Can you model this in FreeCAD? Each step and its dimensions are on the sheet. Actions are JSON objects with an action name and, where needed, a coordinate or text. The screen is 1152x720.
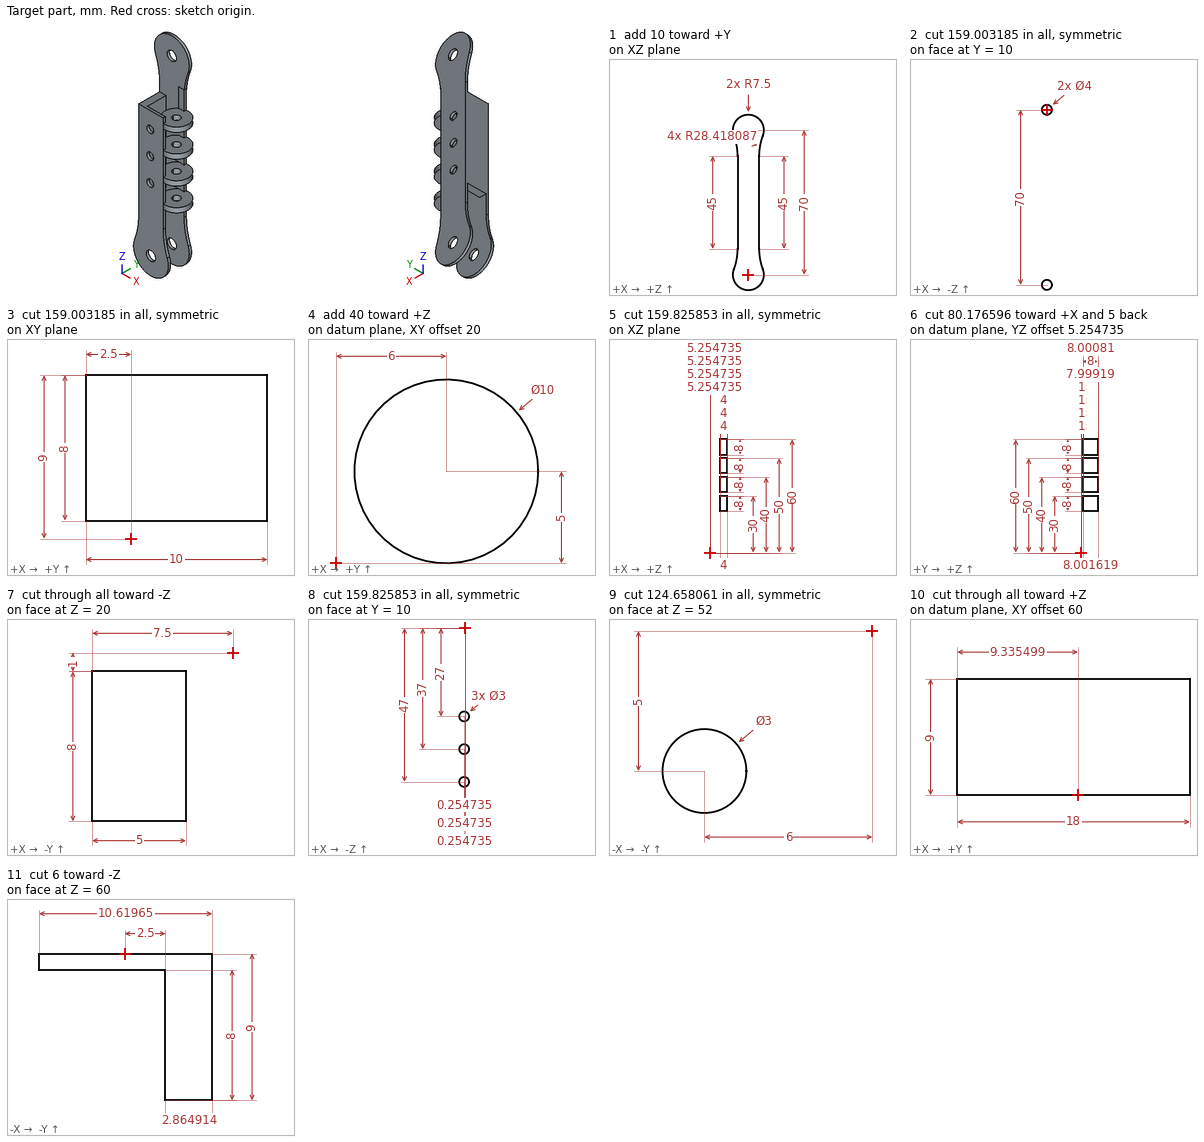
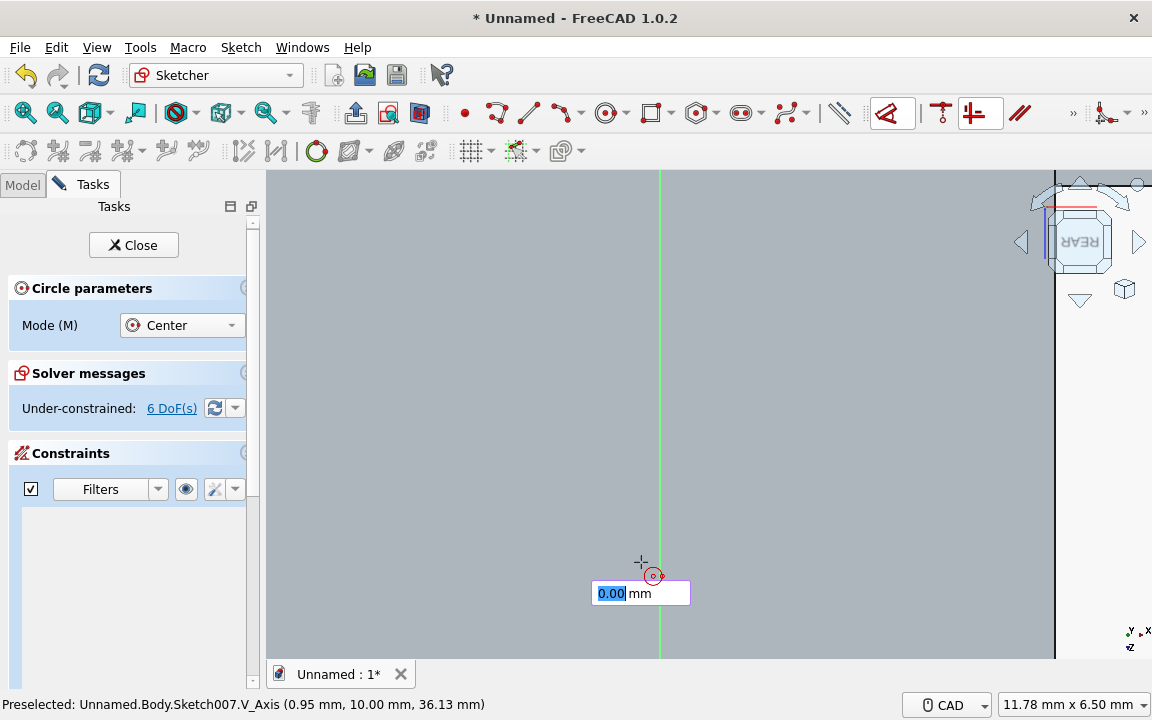
{"action": "scroll", "coordinate": [640, 570], "scroll_direction": "down", "scroll_amount": 12}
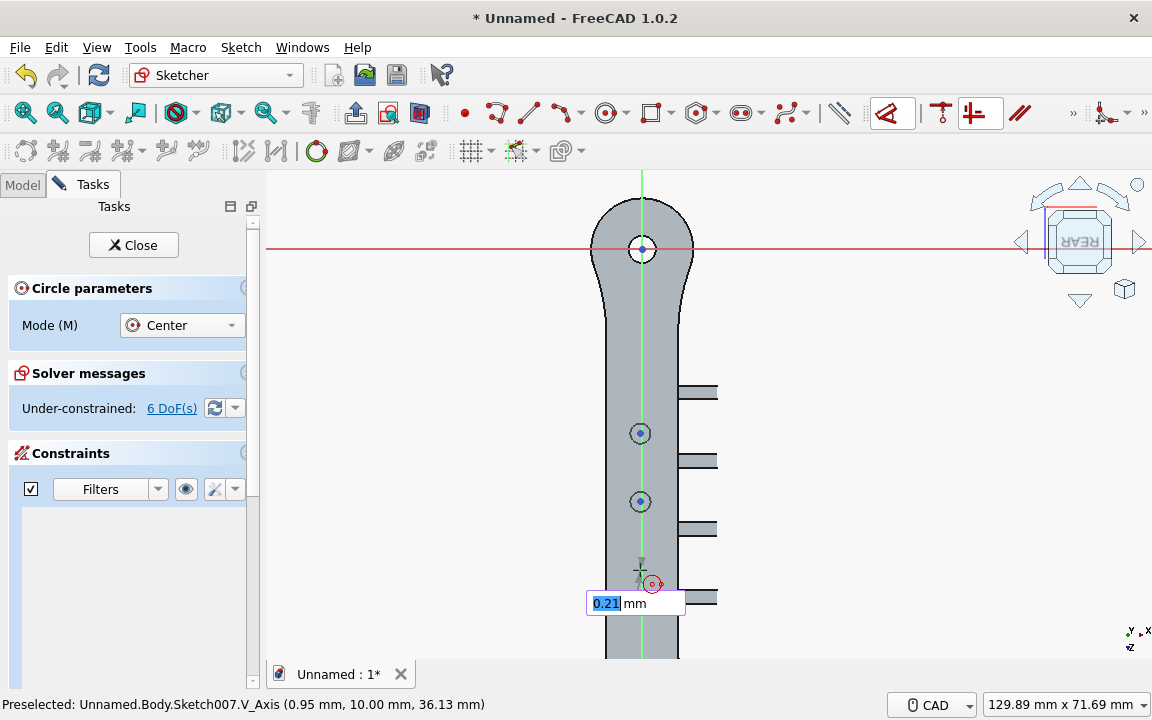
{"action": "scroll", "coordinate": [648, 563], "scroll_direction": "up", "scroll_amount": 6}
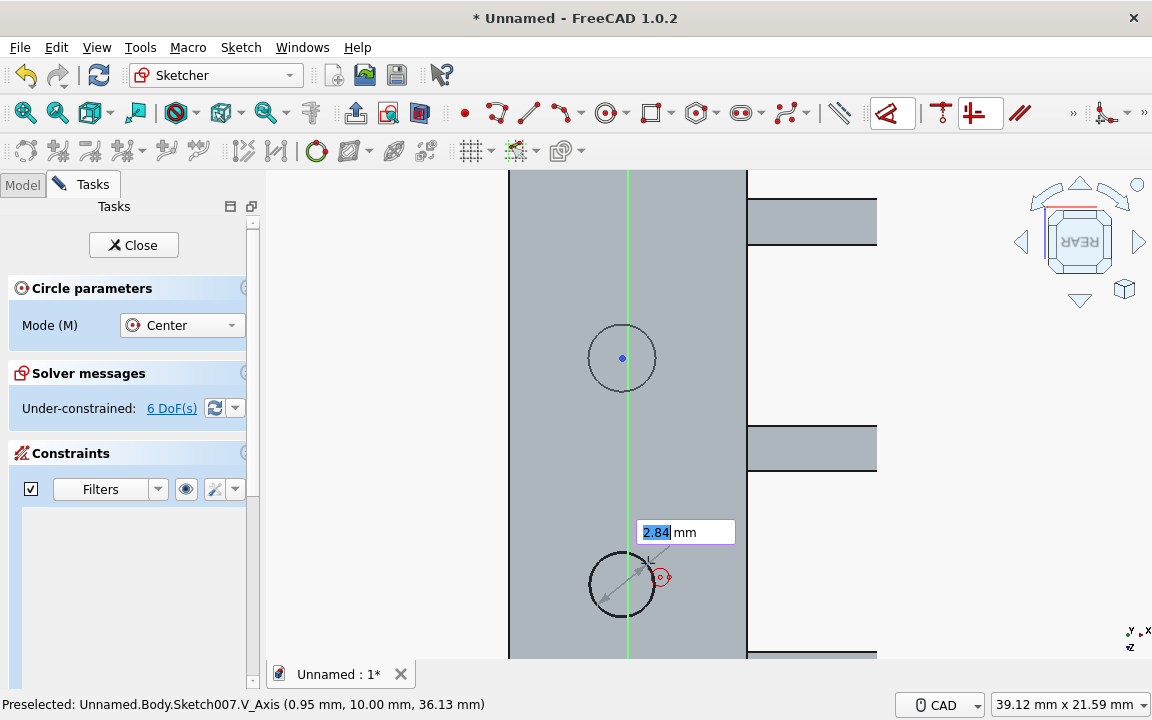
{"action": "left_click", "coordinate": [646, 560]}
{"action": "key", "text": "Escape"}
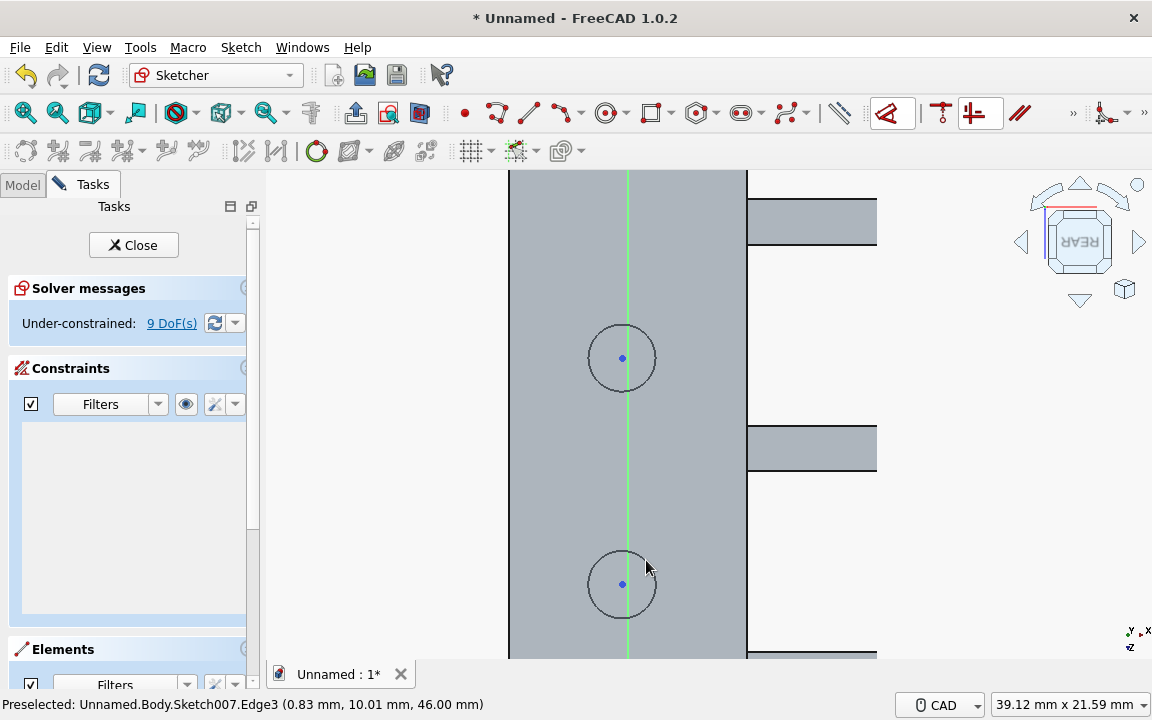
{"action": "scroll", "coordinate": [648, 563], "scroll_direction": "down", "scroll_amount": 6}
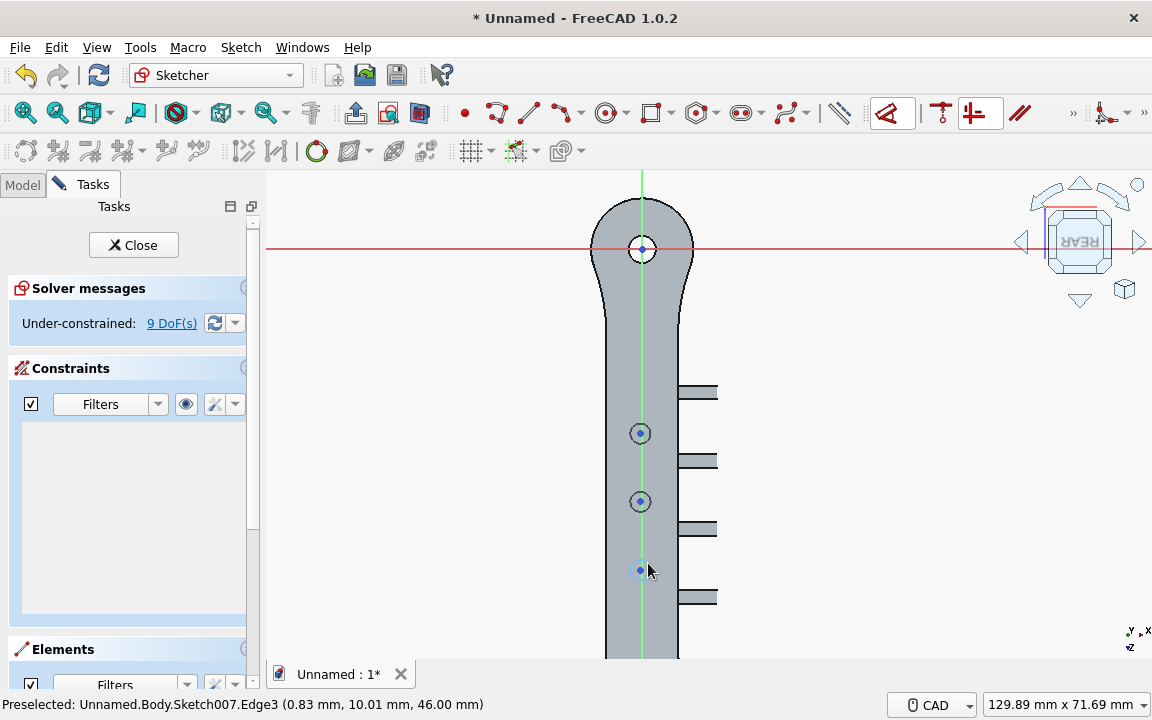
{"action": "scroll", "coordinate": [648, 426], "scroll_direction": "up", "scroll_amount": 5}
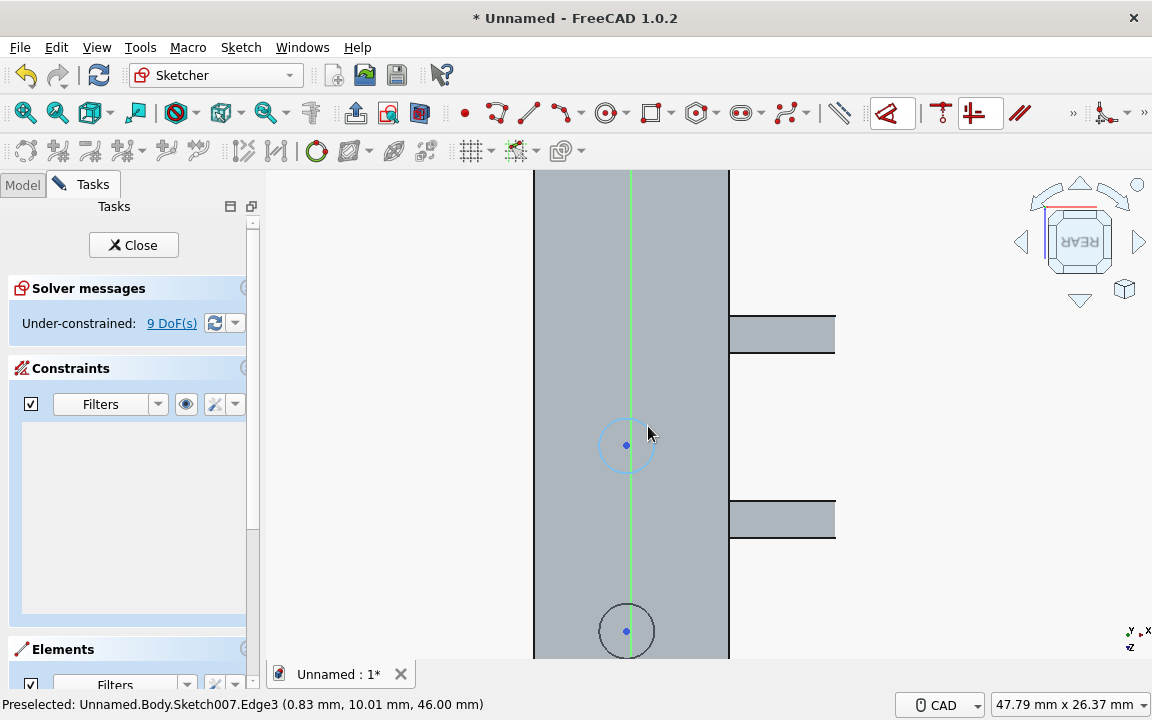
{"action": "left_click", "coordinate": [646, 426]}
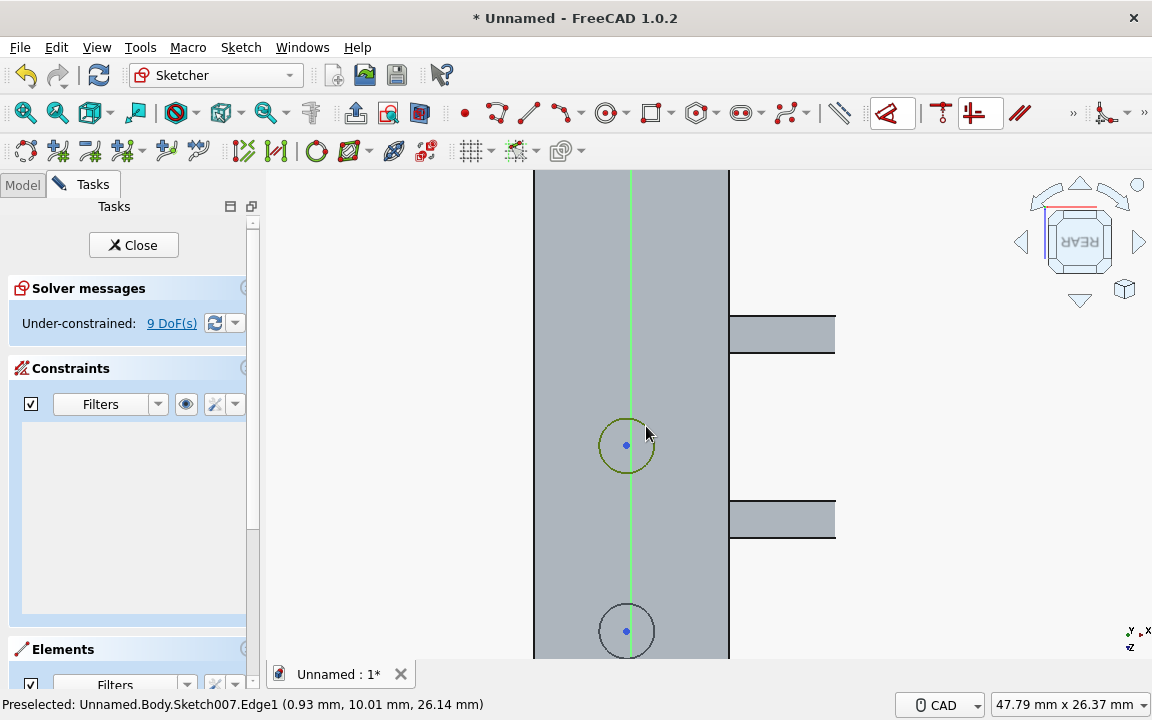
{"action": "left_click", "coordinate": [646, 612]}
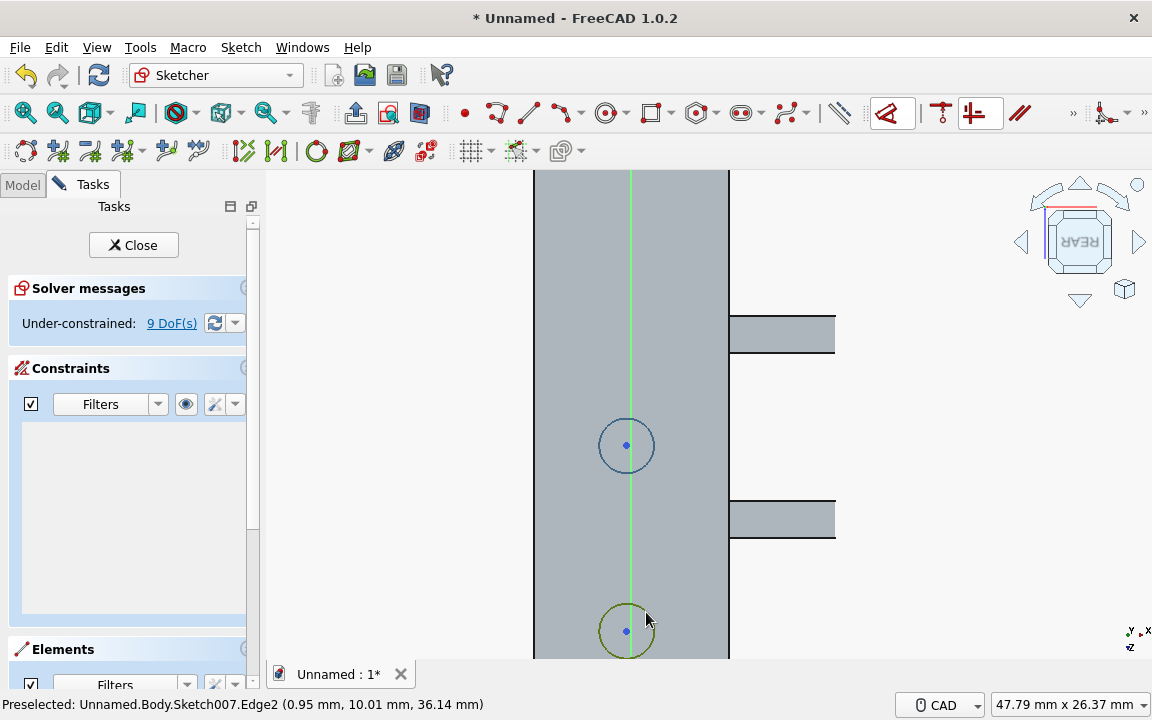
{"action": "scroll", "coordinate": [649, 426], "scroll_direction": "down", "scroll_amount": 5}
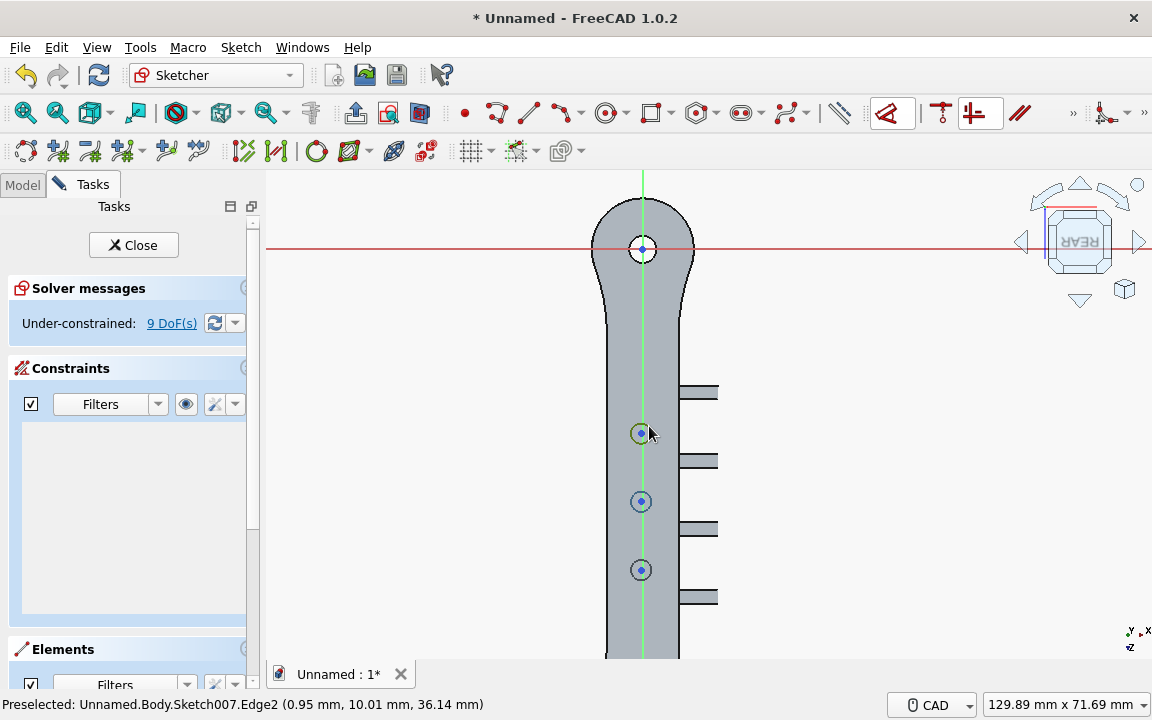
{"action": "scroll", "coordinate": [648, 563], "scroll_direction": "up", "scroll_amount": 5}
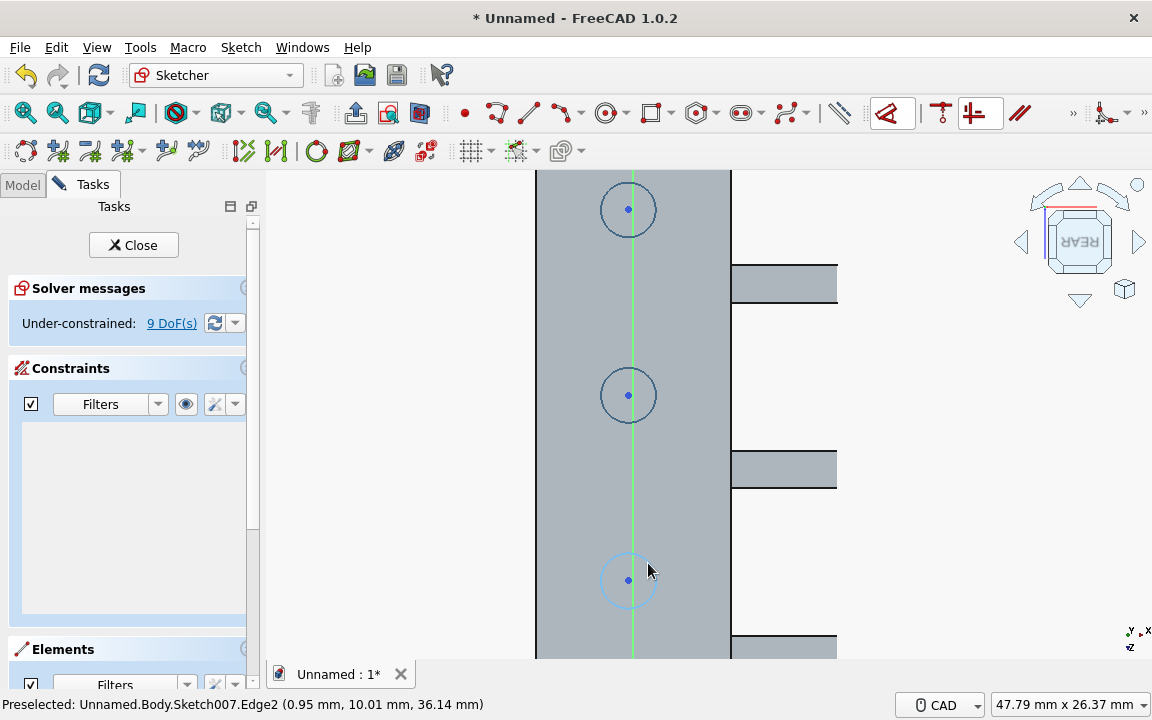
{"action": "left_click", "coordinate": [648, 561]}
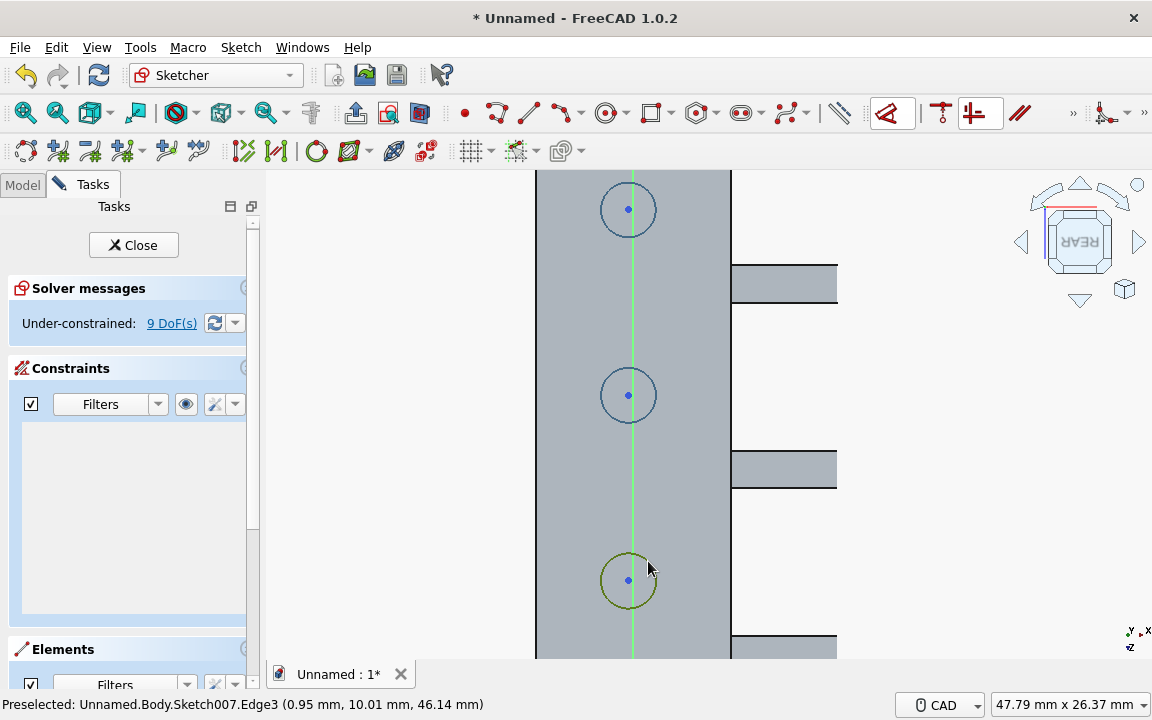
{"action": "key", "text": "e"}